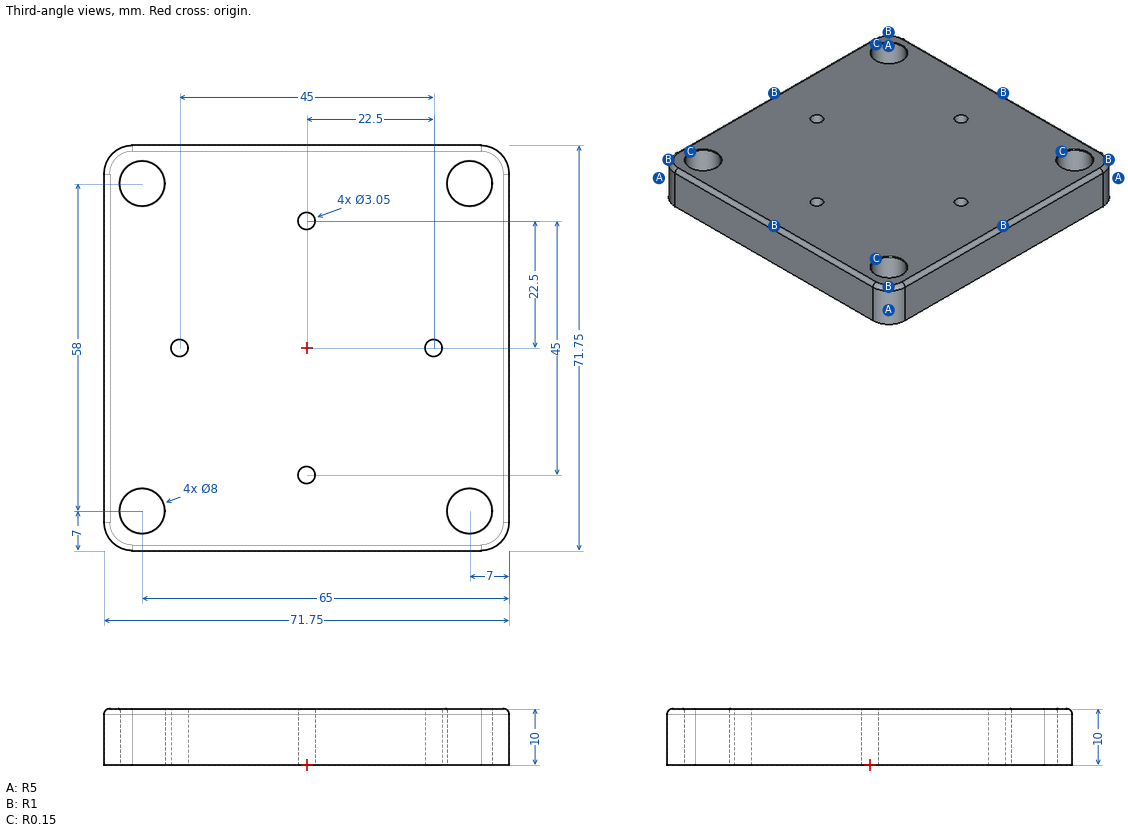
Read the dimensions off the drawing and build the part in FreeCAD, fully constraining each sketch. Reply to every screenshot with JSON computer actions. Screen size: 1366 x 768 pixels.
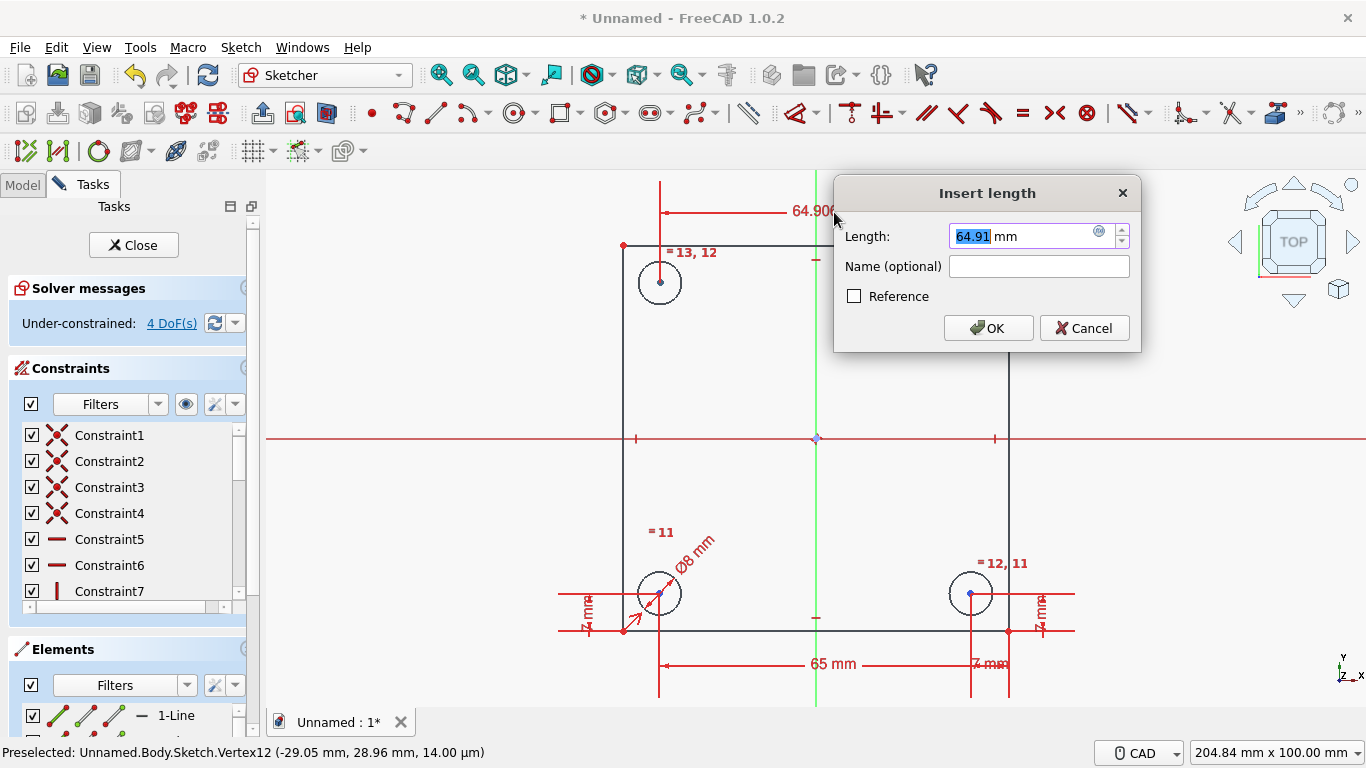
{"action": "type", "text": "65"}
{"action": "key", "text": "Return"}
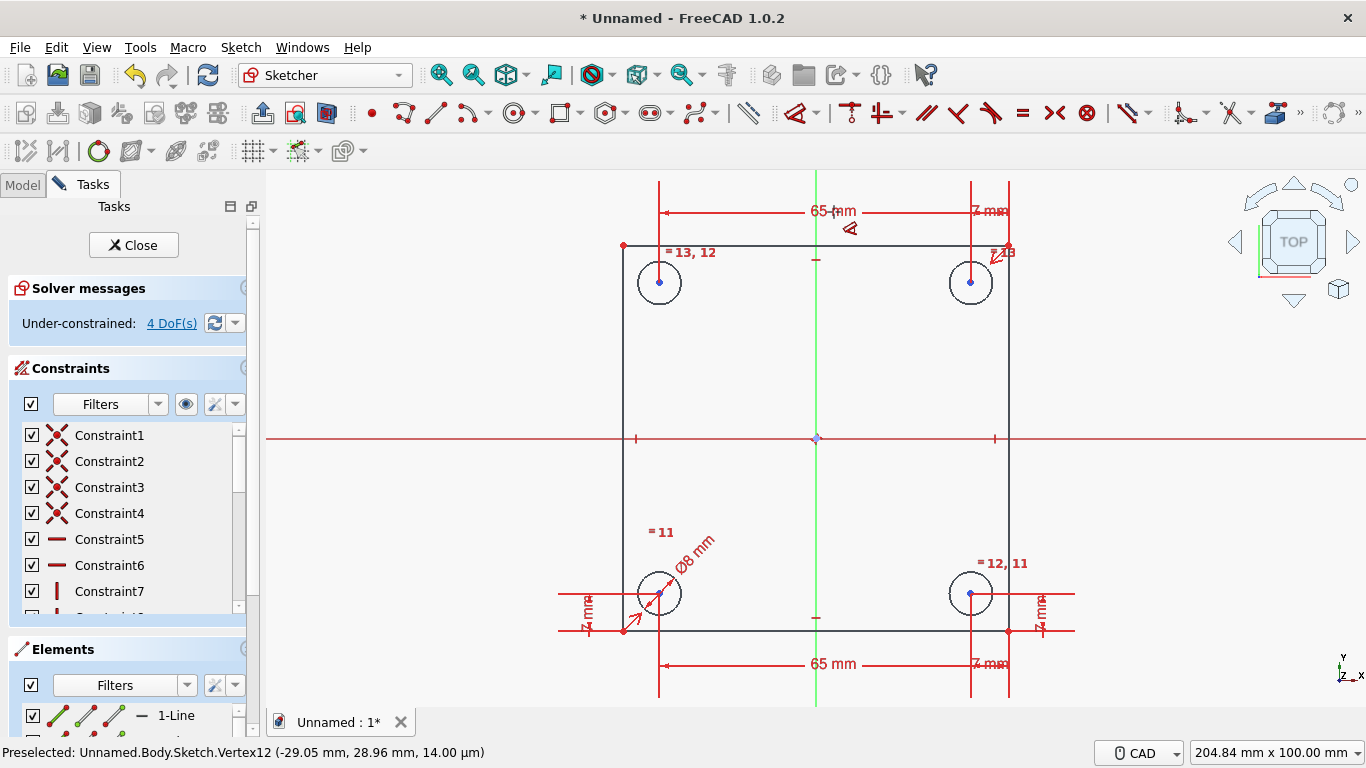
{"action": "left_click", "coordinate": [659, 594]}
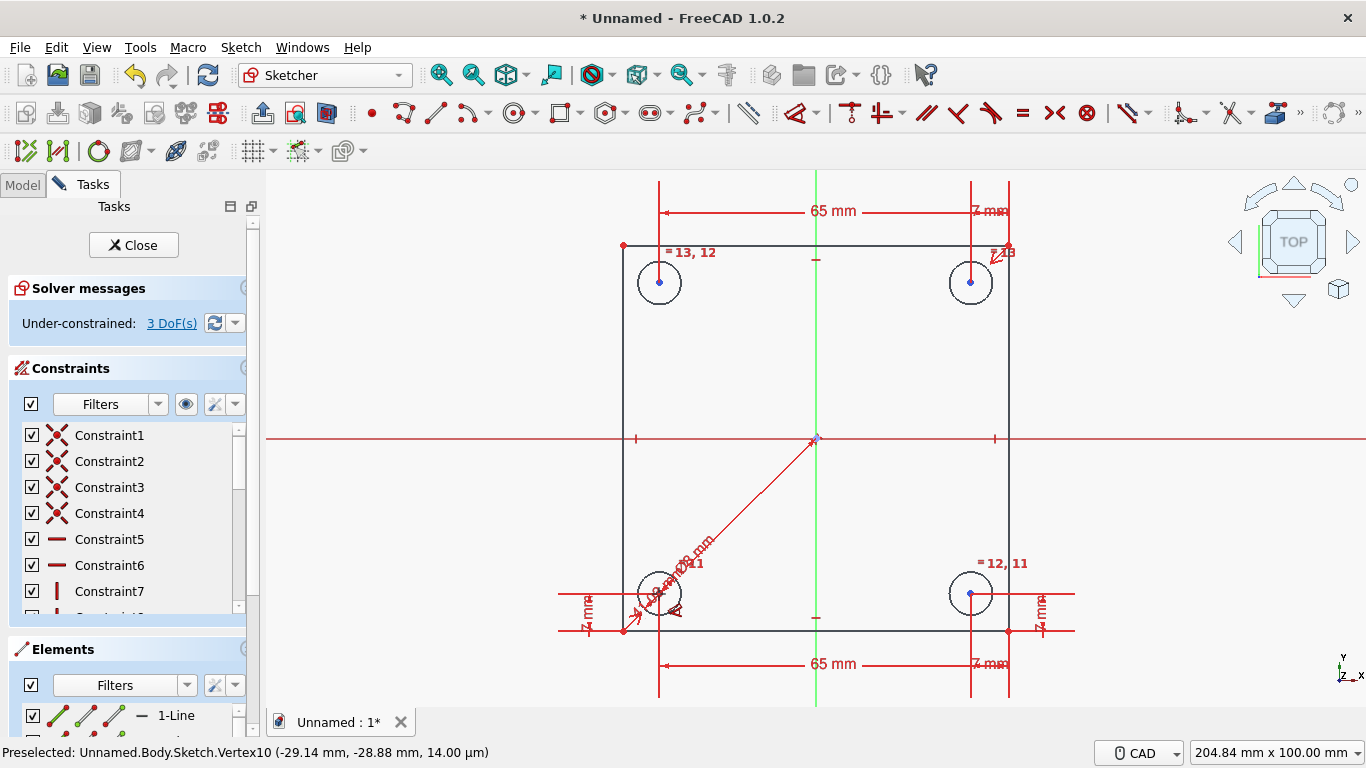
{"action": "left_click", "coordinate": [659, 283]}
{"action": "left_click", "coordinate": [693, 367]}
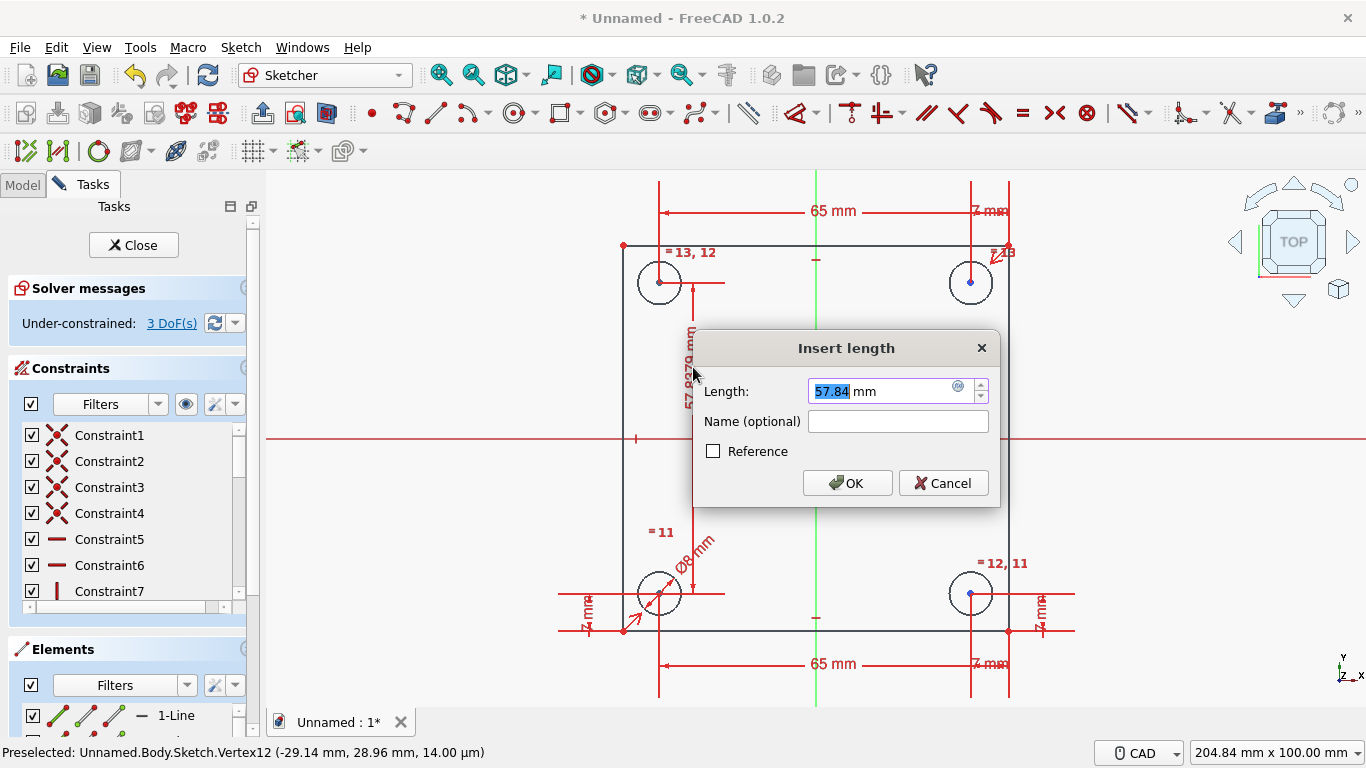
{"action": "type", "text": "58"}
{"action": "key", "text": "Return"}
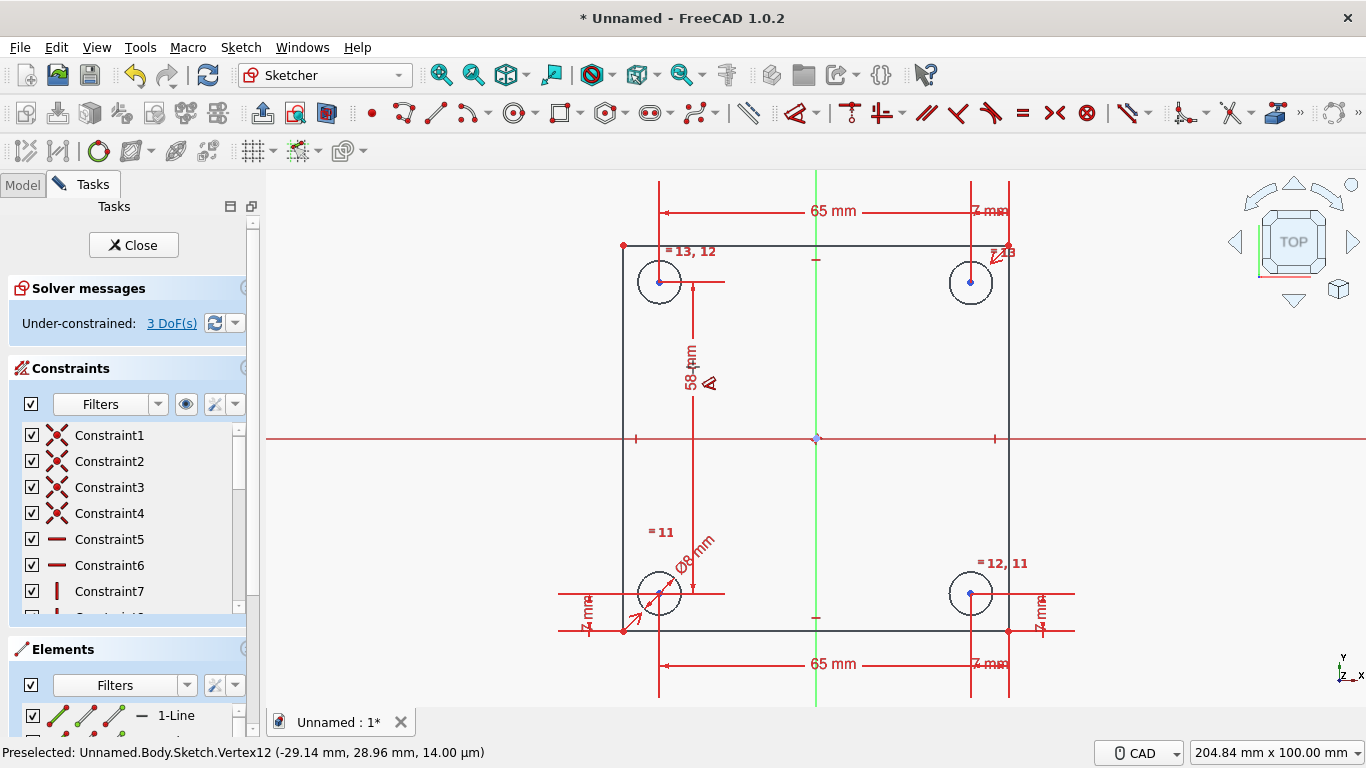
{"action": "left_click", "coordinate": [971, 594]}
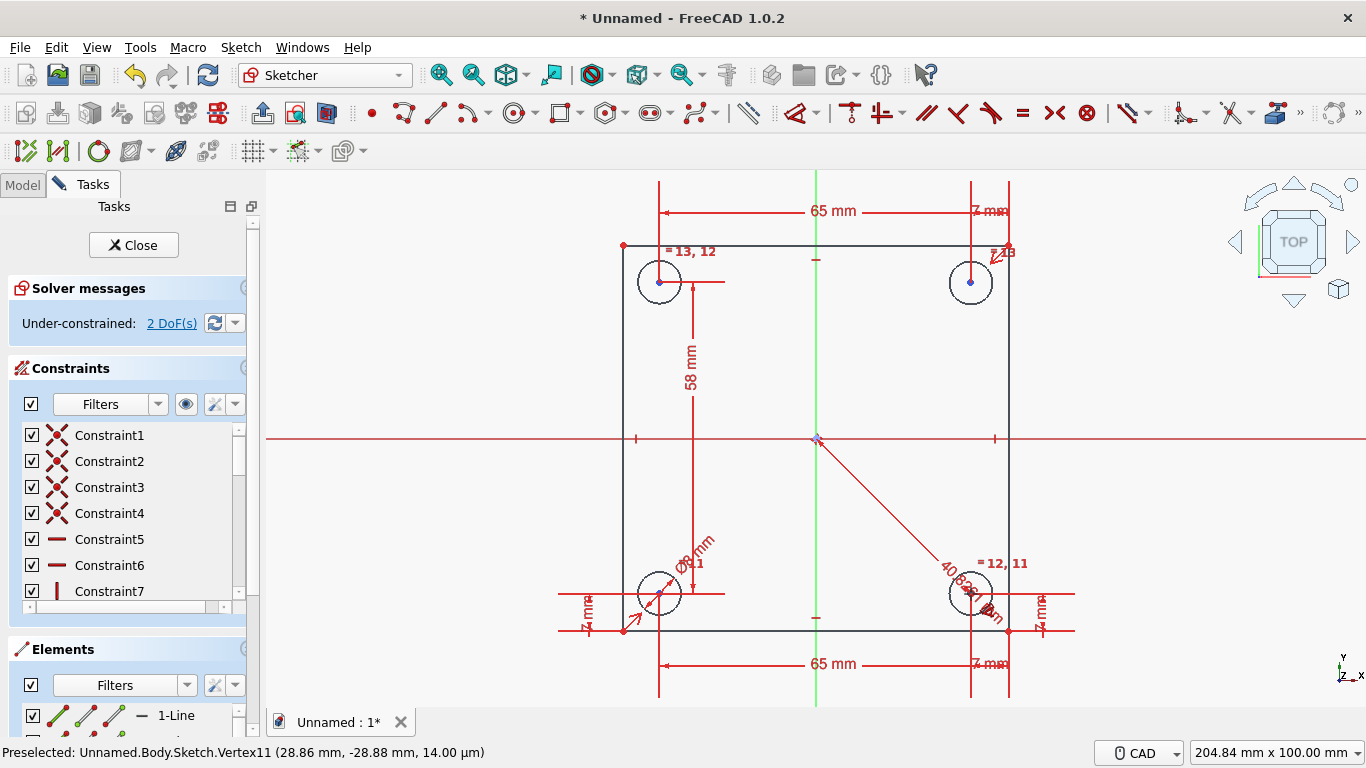
{"action": "left_click", "coordinate": [971, 283]}
{"action": "left_click", "coordinate": [937, 367]}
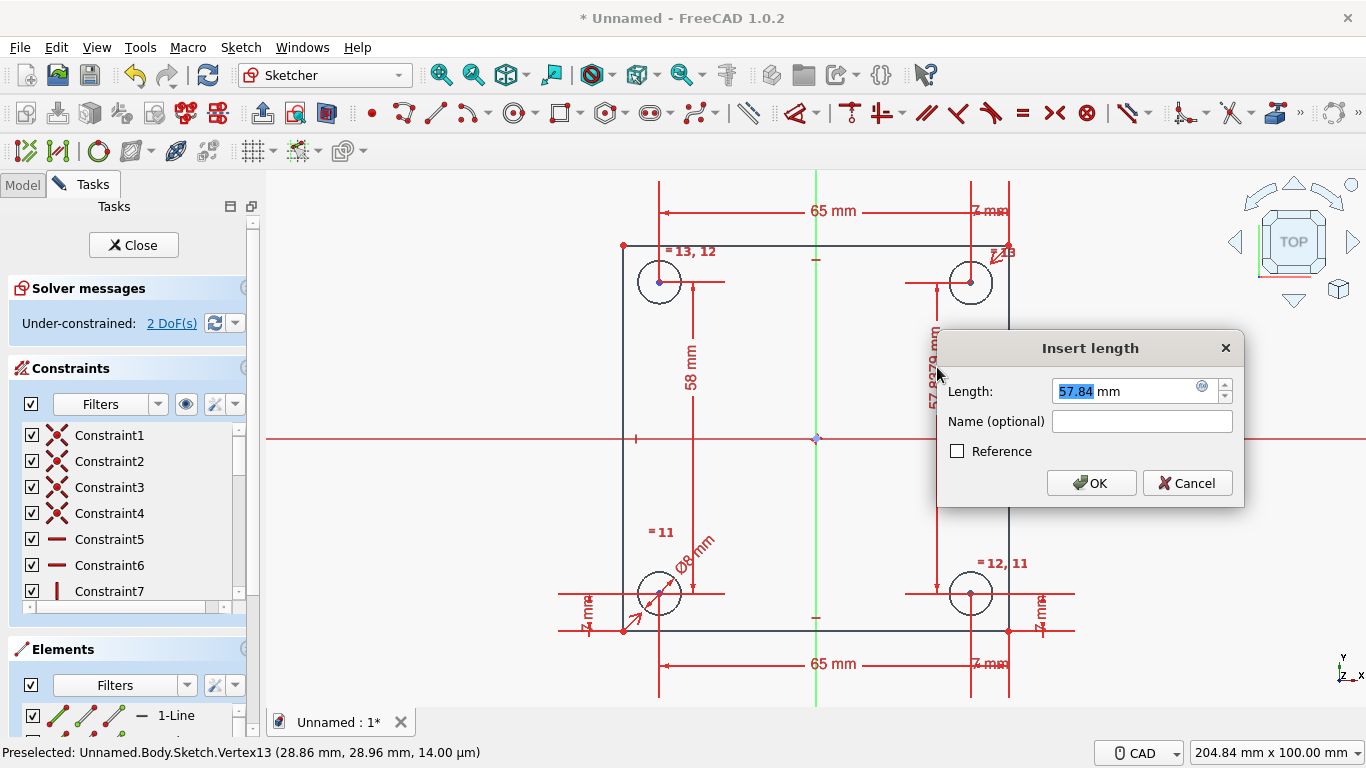
{"action": "type", "text": "58"}
{"action": "key", "text": "Return"}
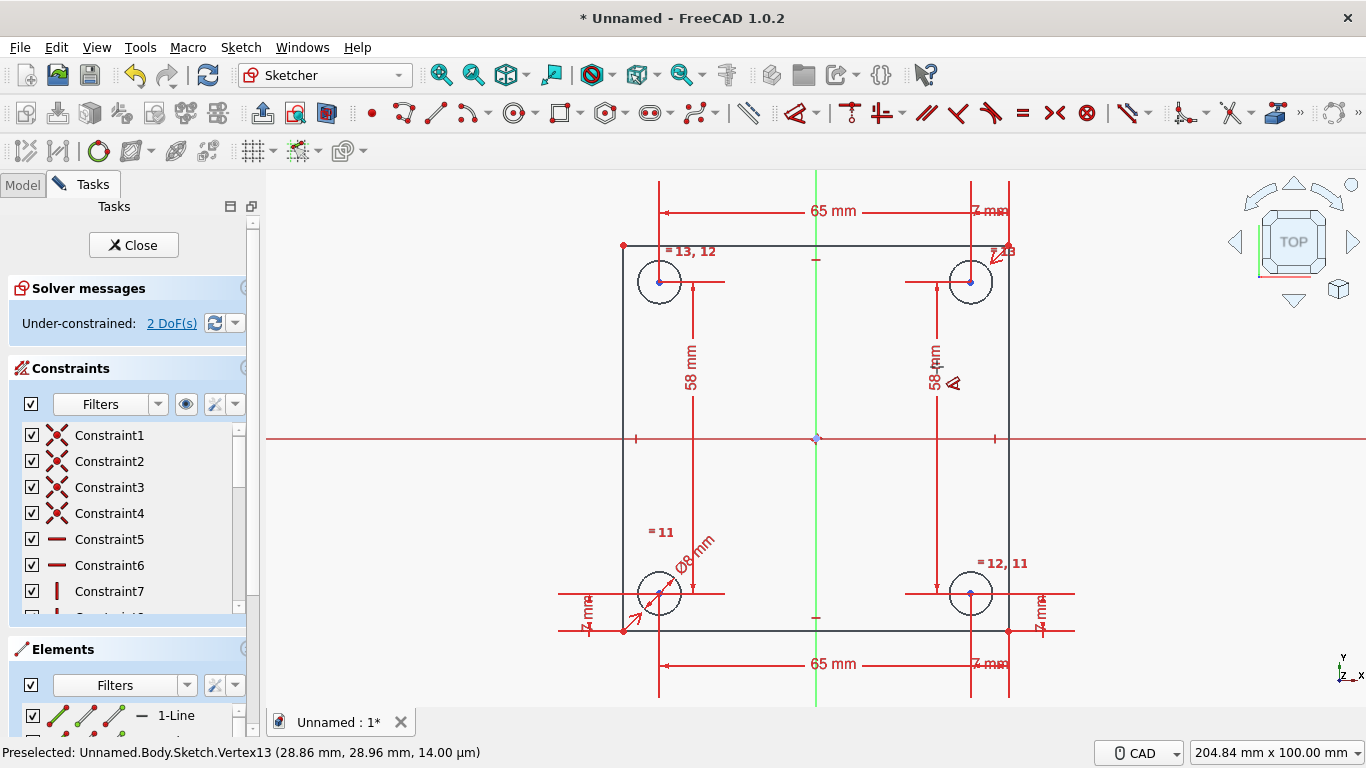
{"action": "left_click", "coordinate": [739, 631]}
{"action": "left_click", "coordinate": [727, 665]}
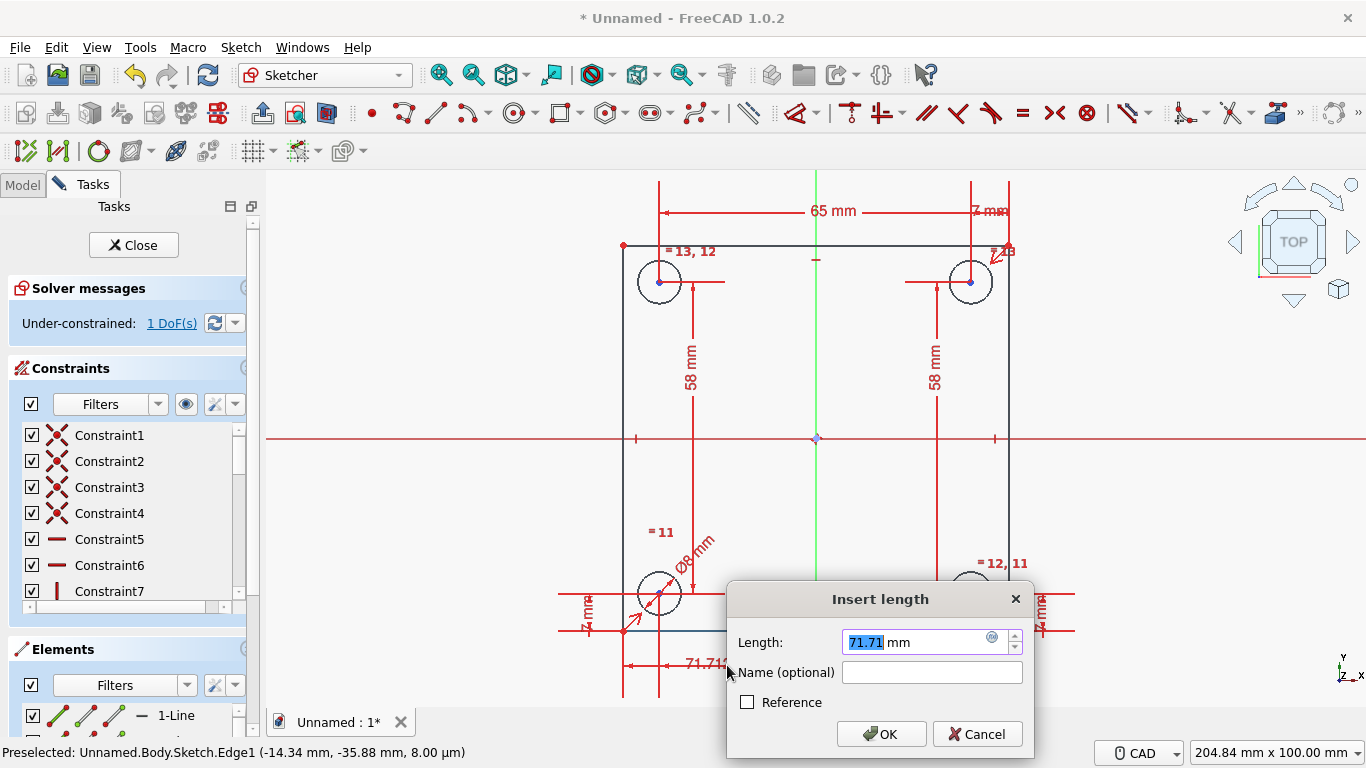
{"action": "type", "text": "71.75"}
{"action": "key", "text": "Return"}